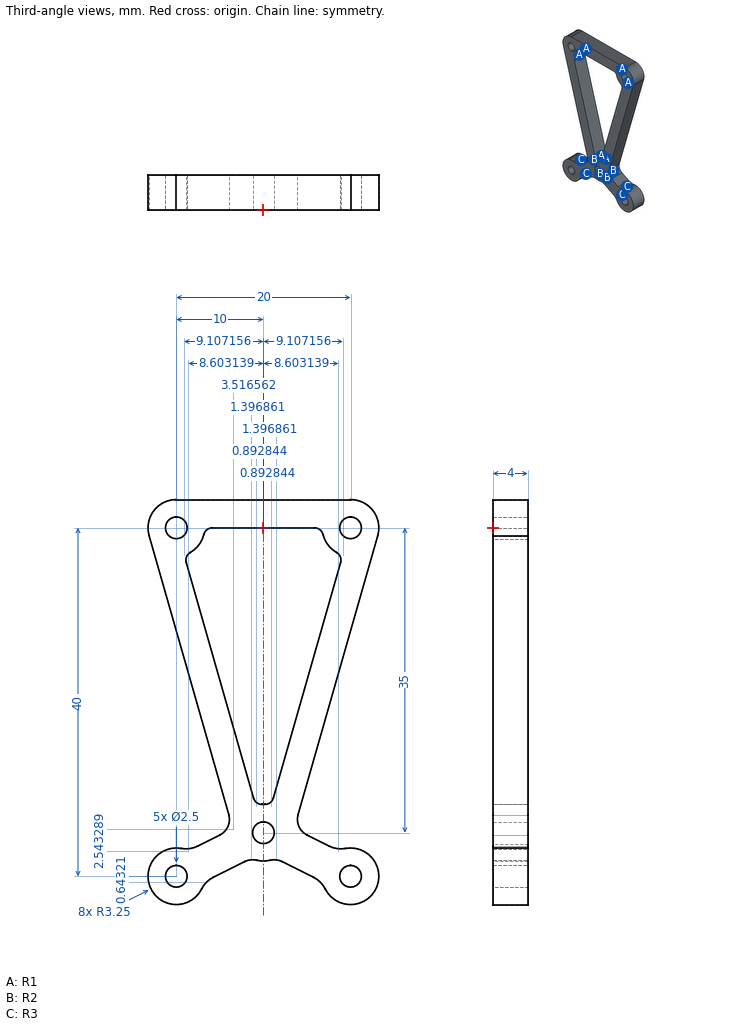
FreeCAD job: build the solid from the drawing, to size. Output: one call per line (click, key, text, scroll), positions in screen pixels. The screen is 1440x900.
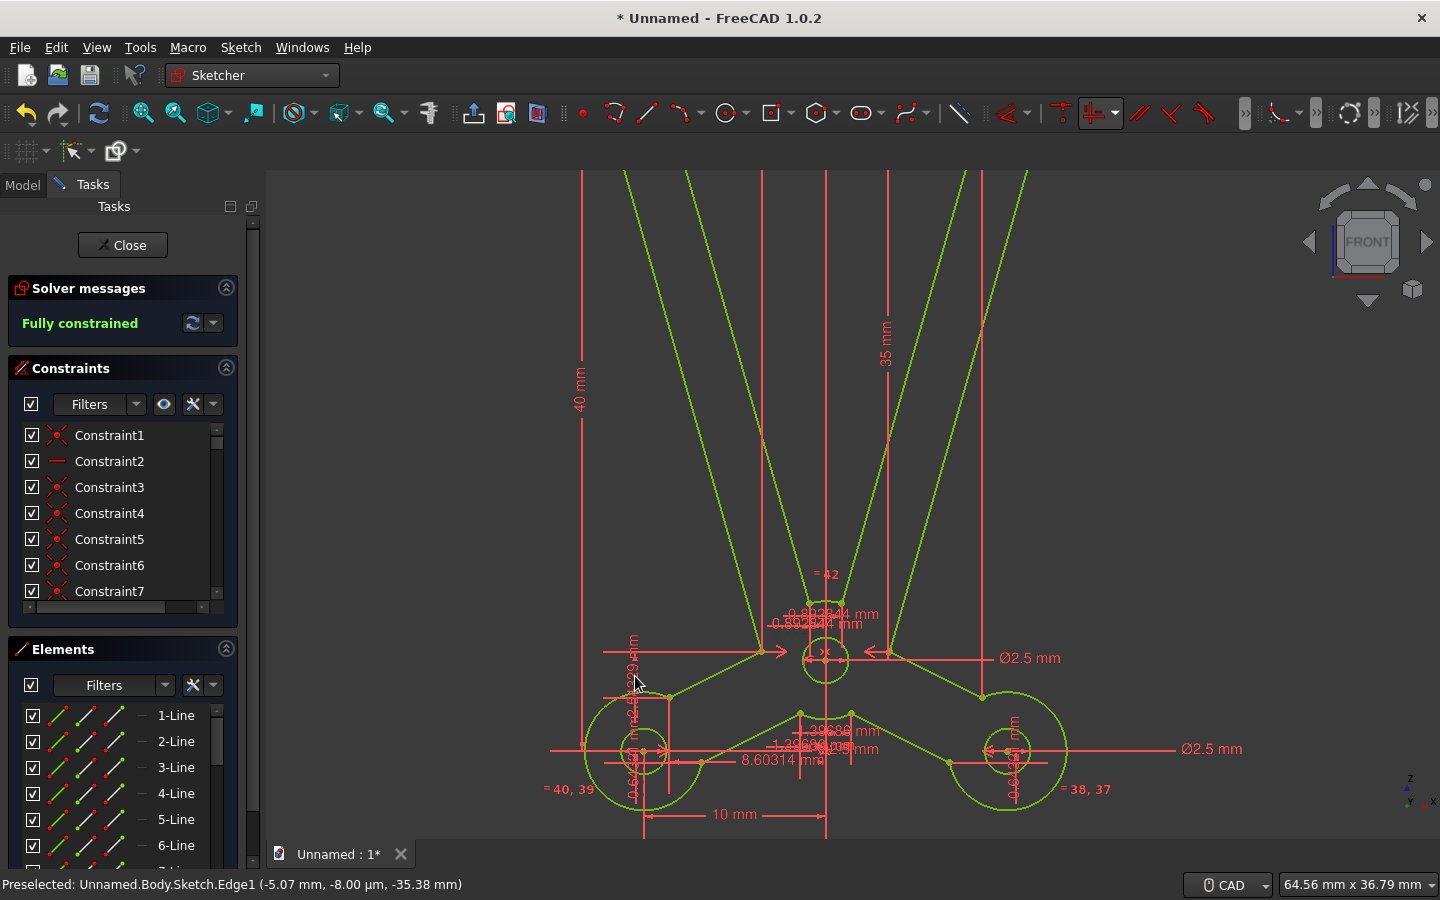
click(123, 245)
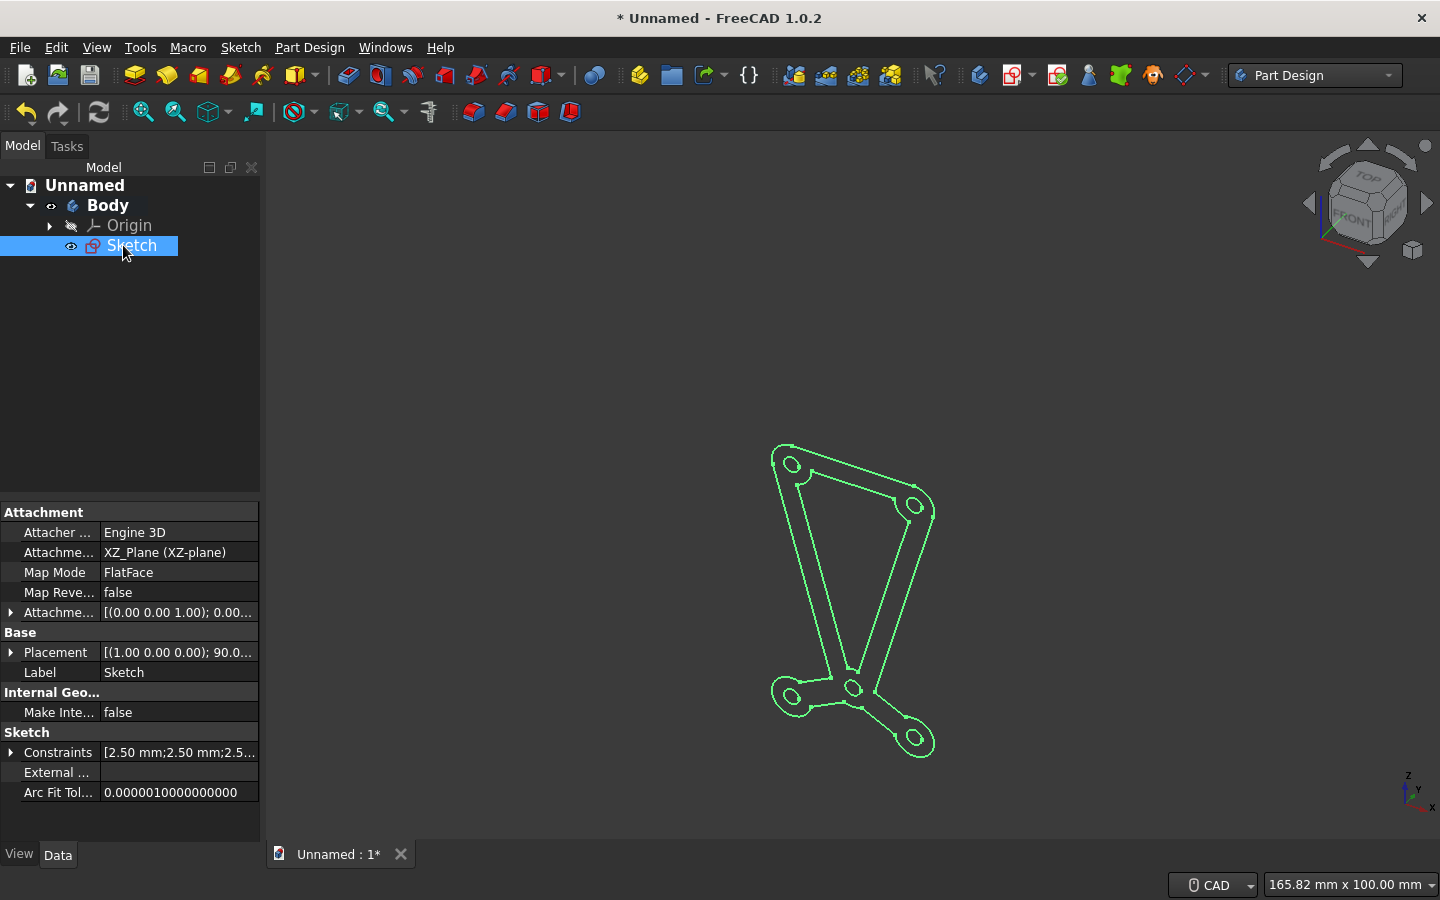
click(136, 76)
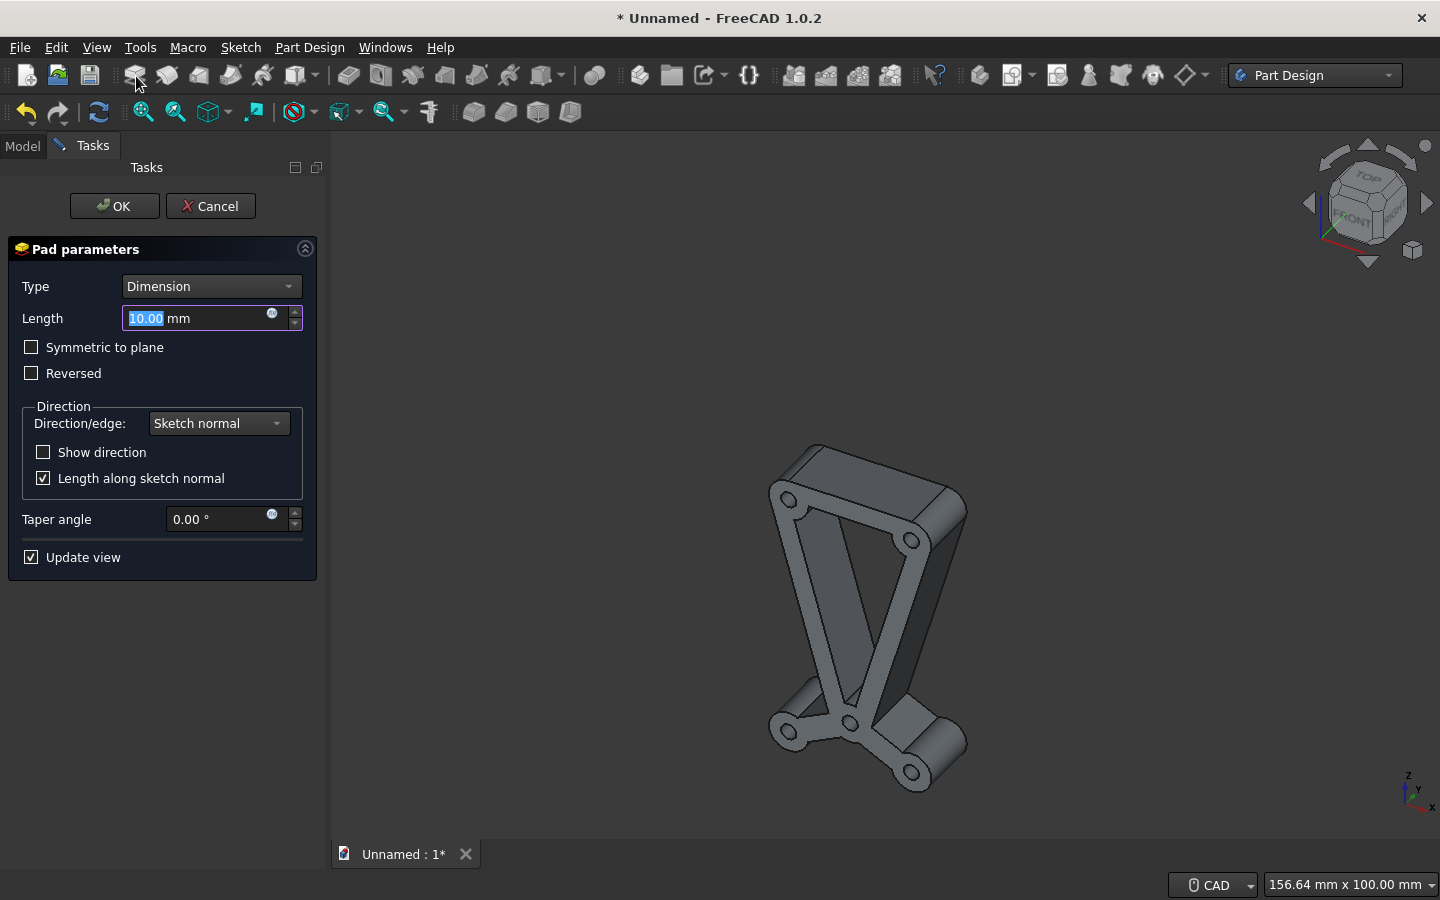
text(4)
key(Tab)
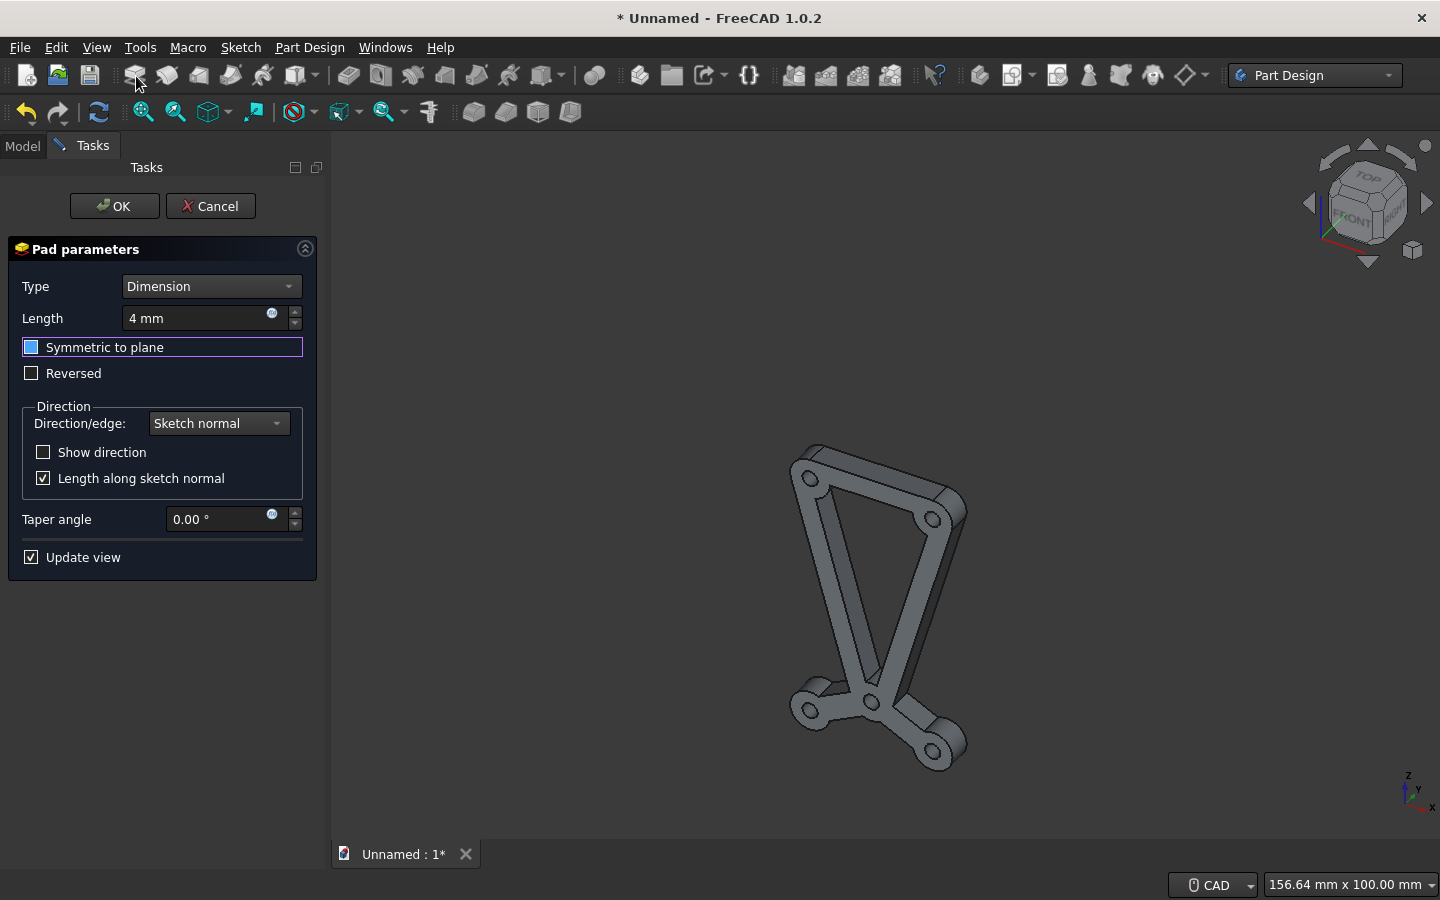
click(30, 373)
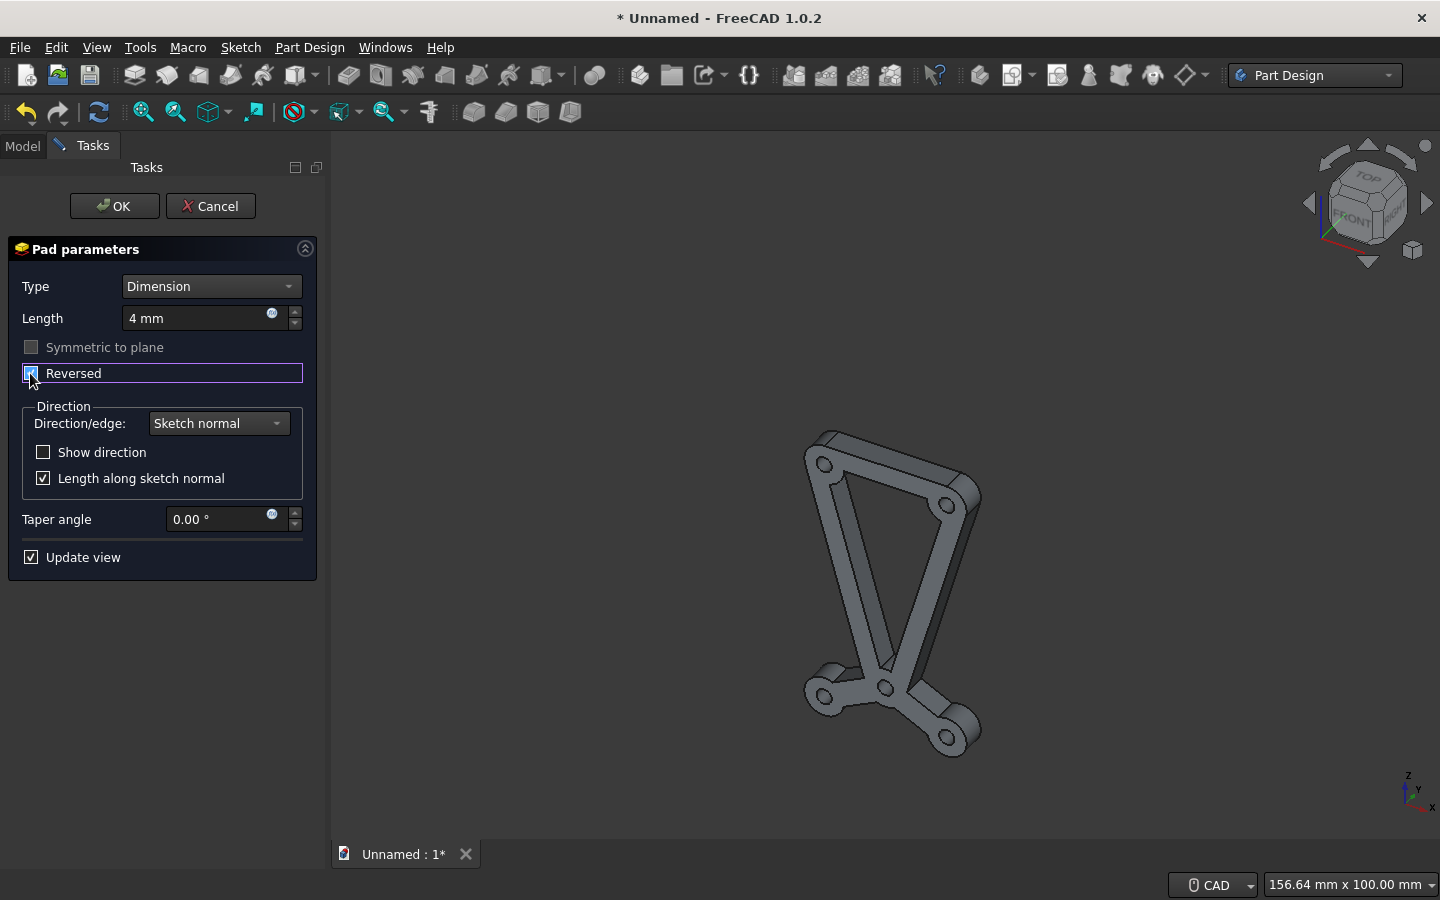
click(115, 206)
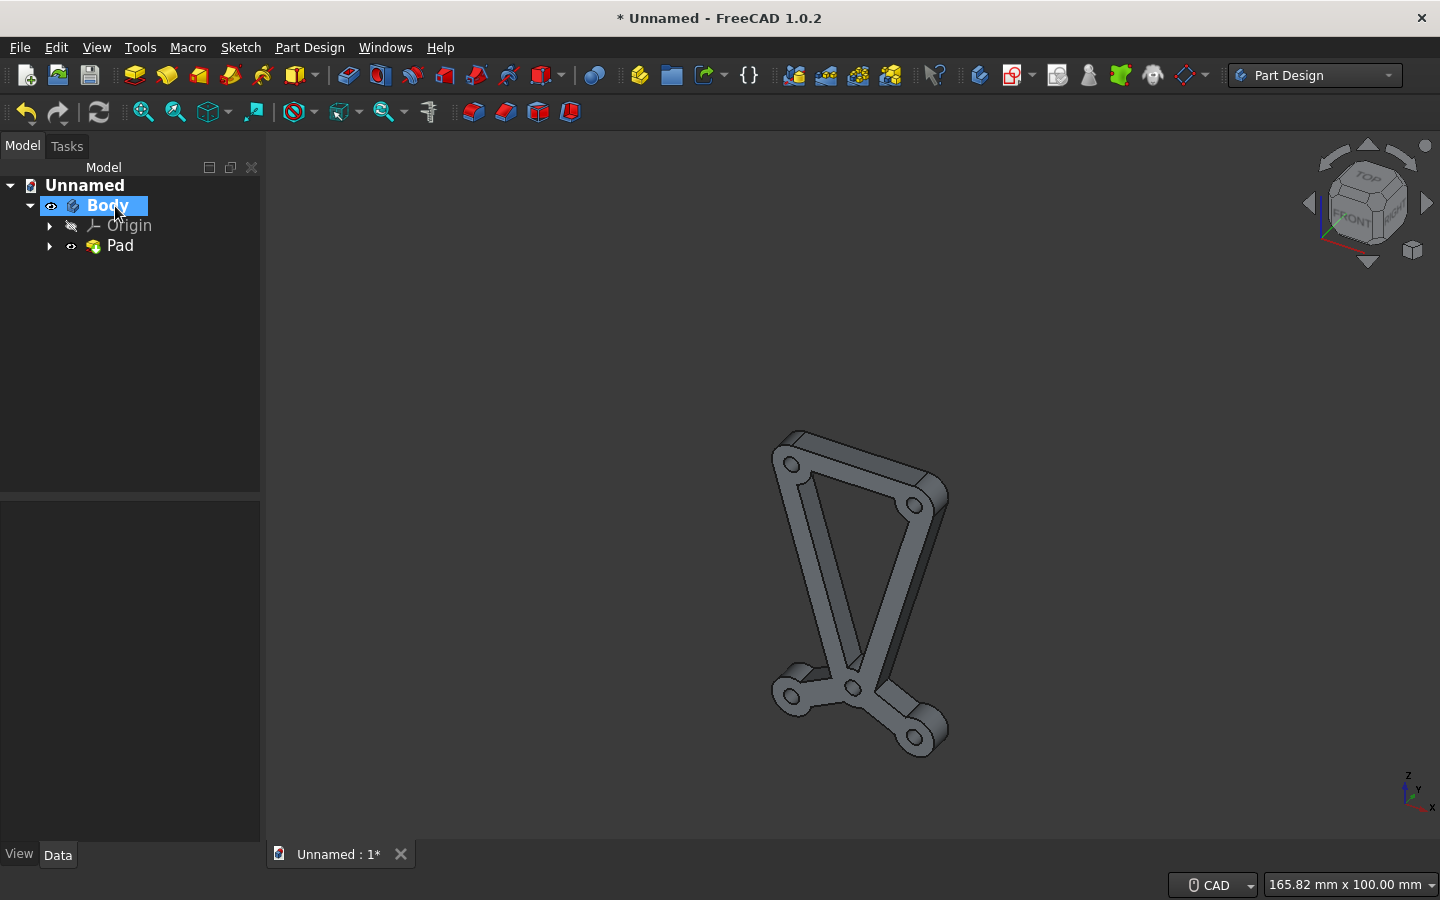
key(0)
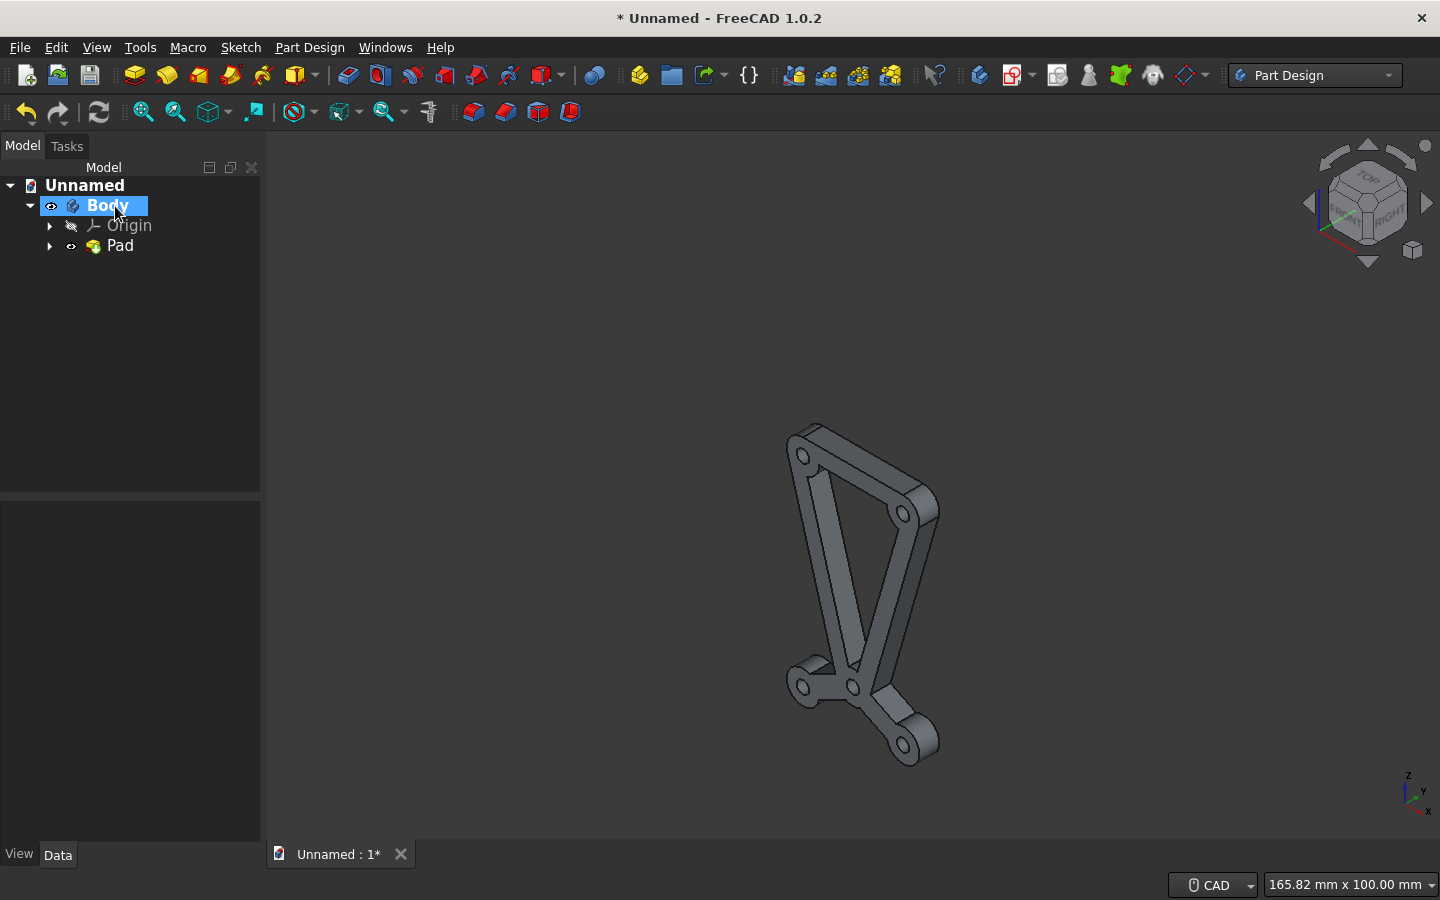
key(2)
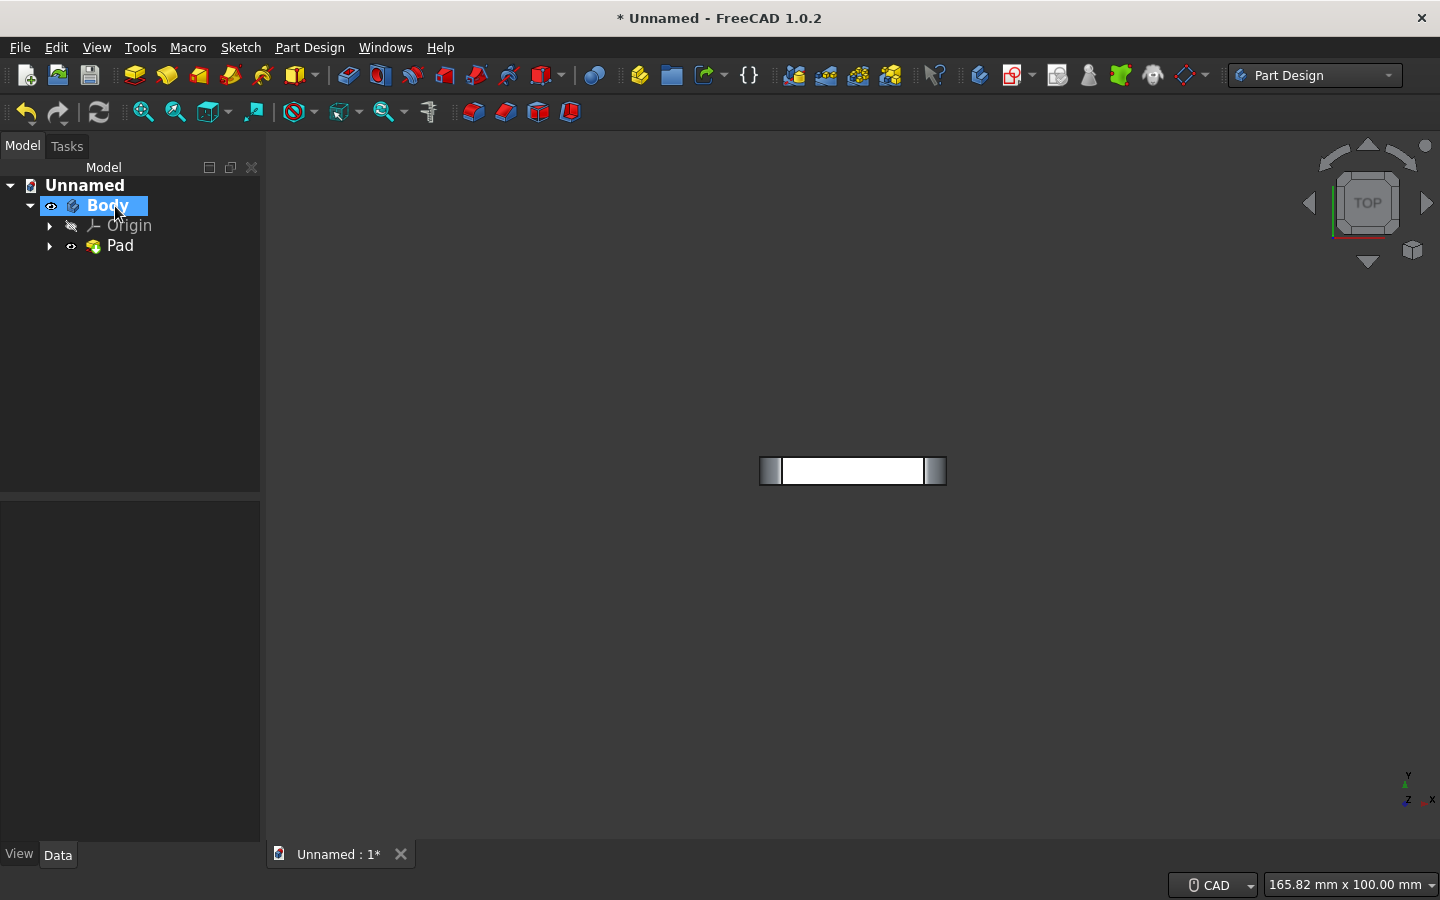
click(144, 112)